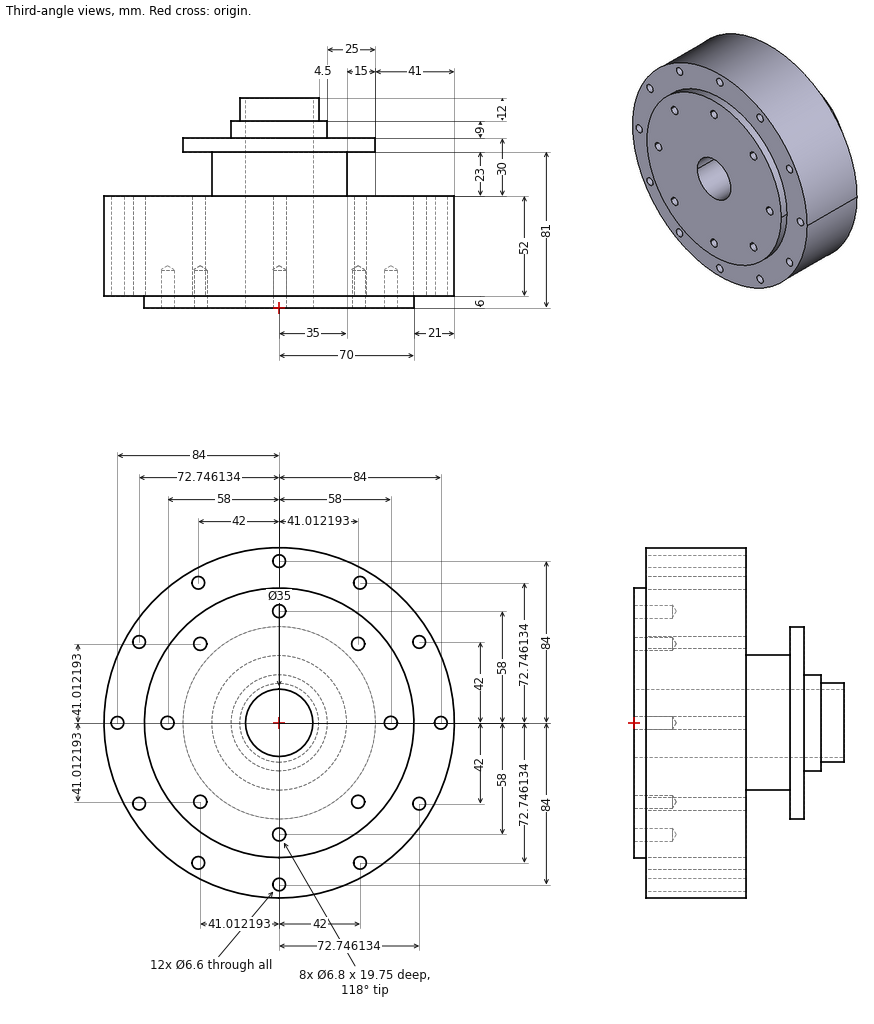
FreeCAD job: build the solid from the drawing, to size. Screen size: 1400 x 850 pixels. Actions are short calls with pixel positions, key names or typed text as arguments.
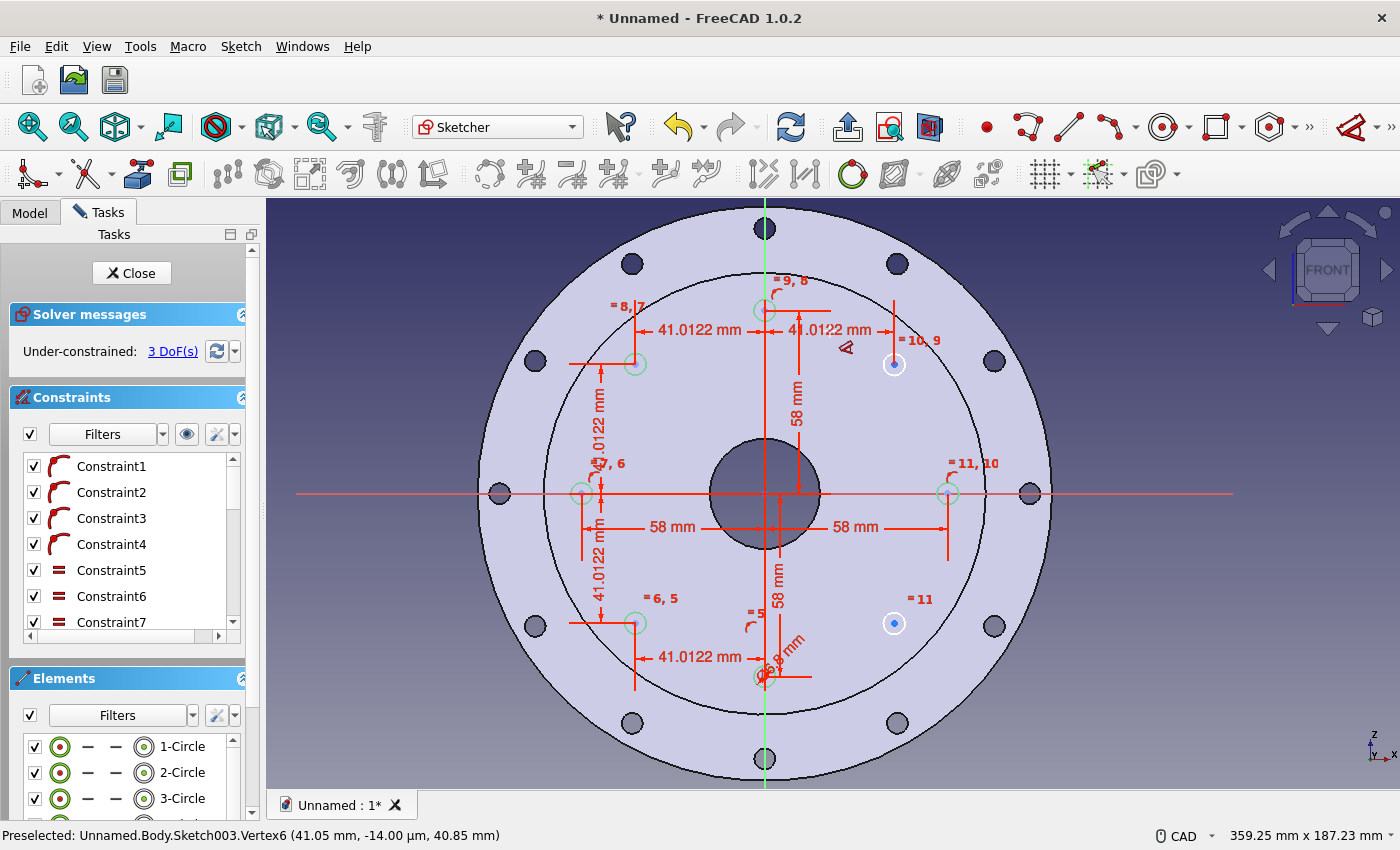
click(894, 365)
click(928, 429)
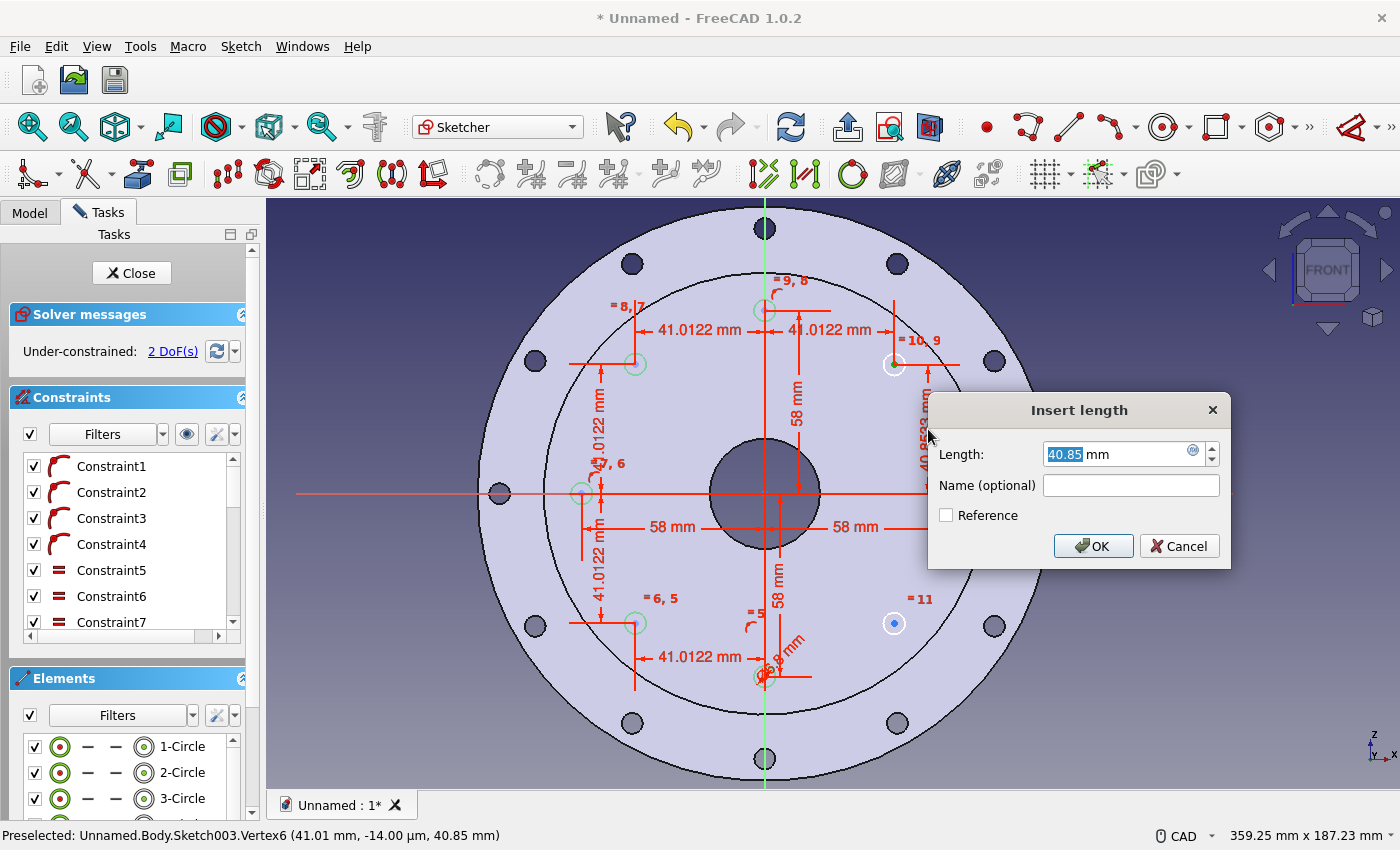
text(41.012193)
key(Return)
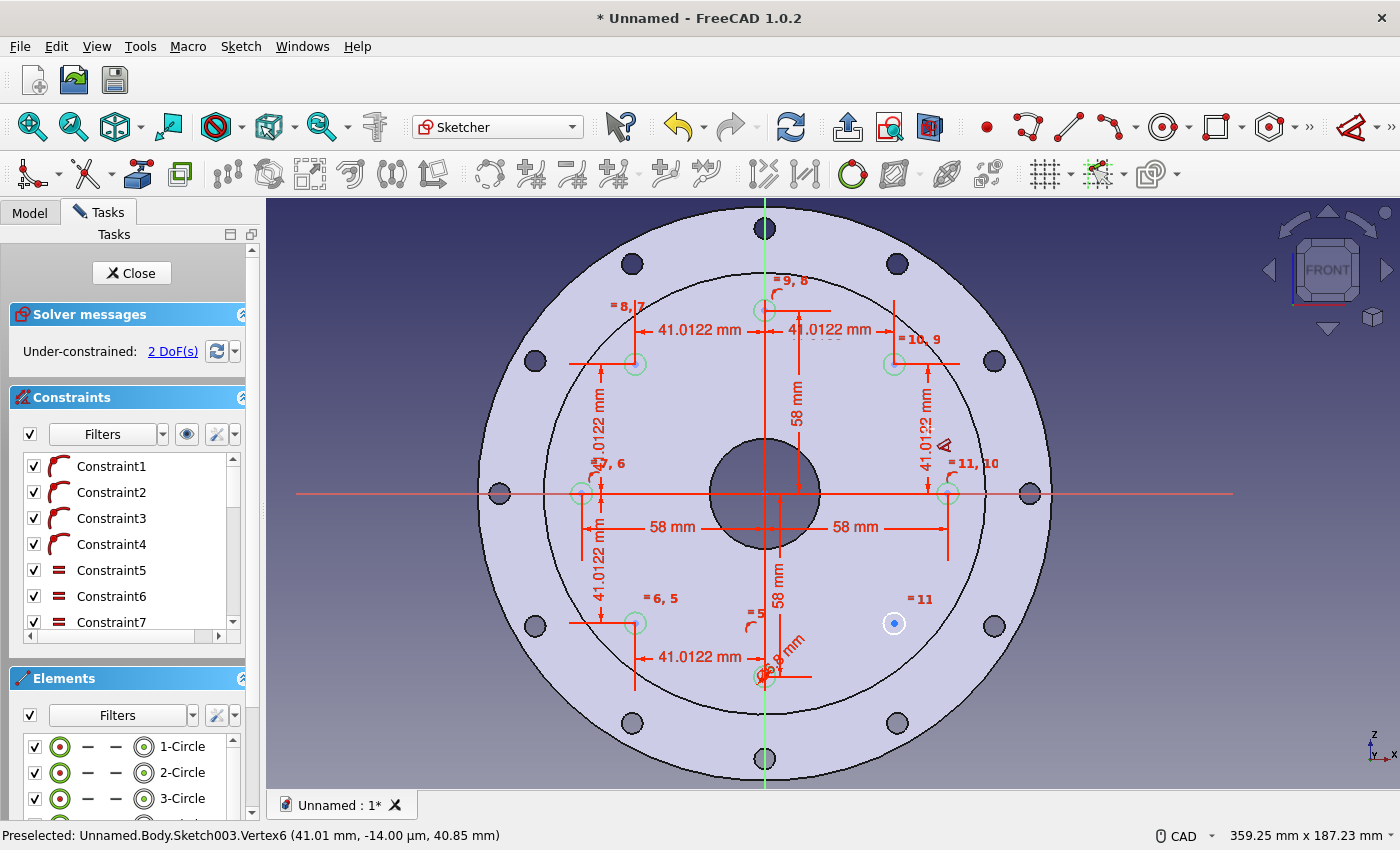
click(894, 624)
click(859, 658)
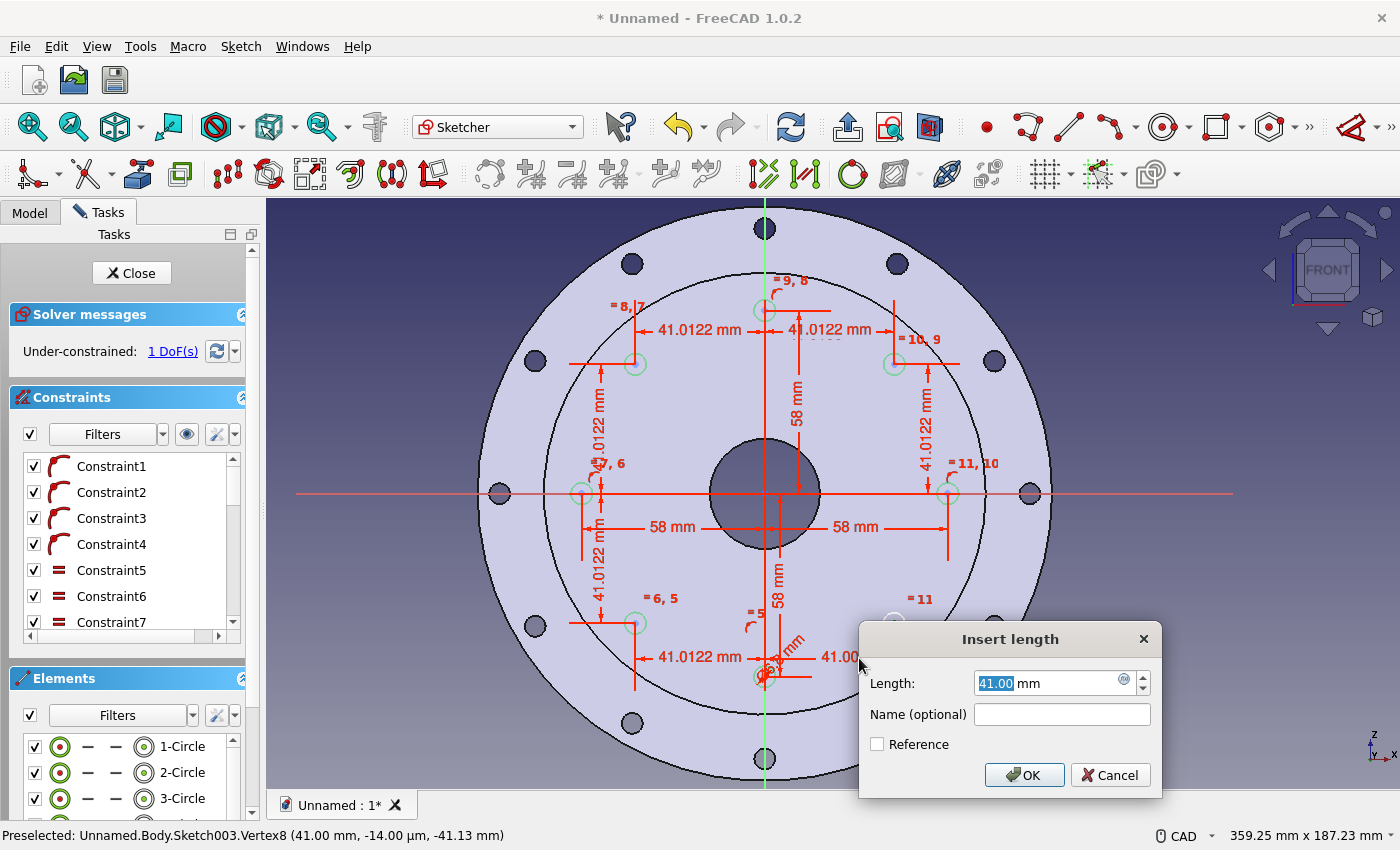
text(41.012193)
key(Return)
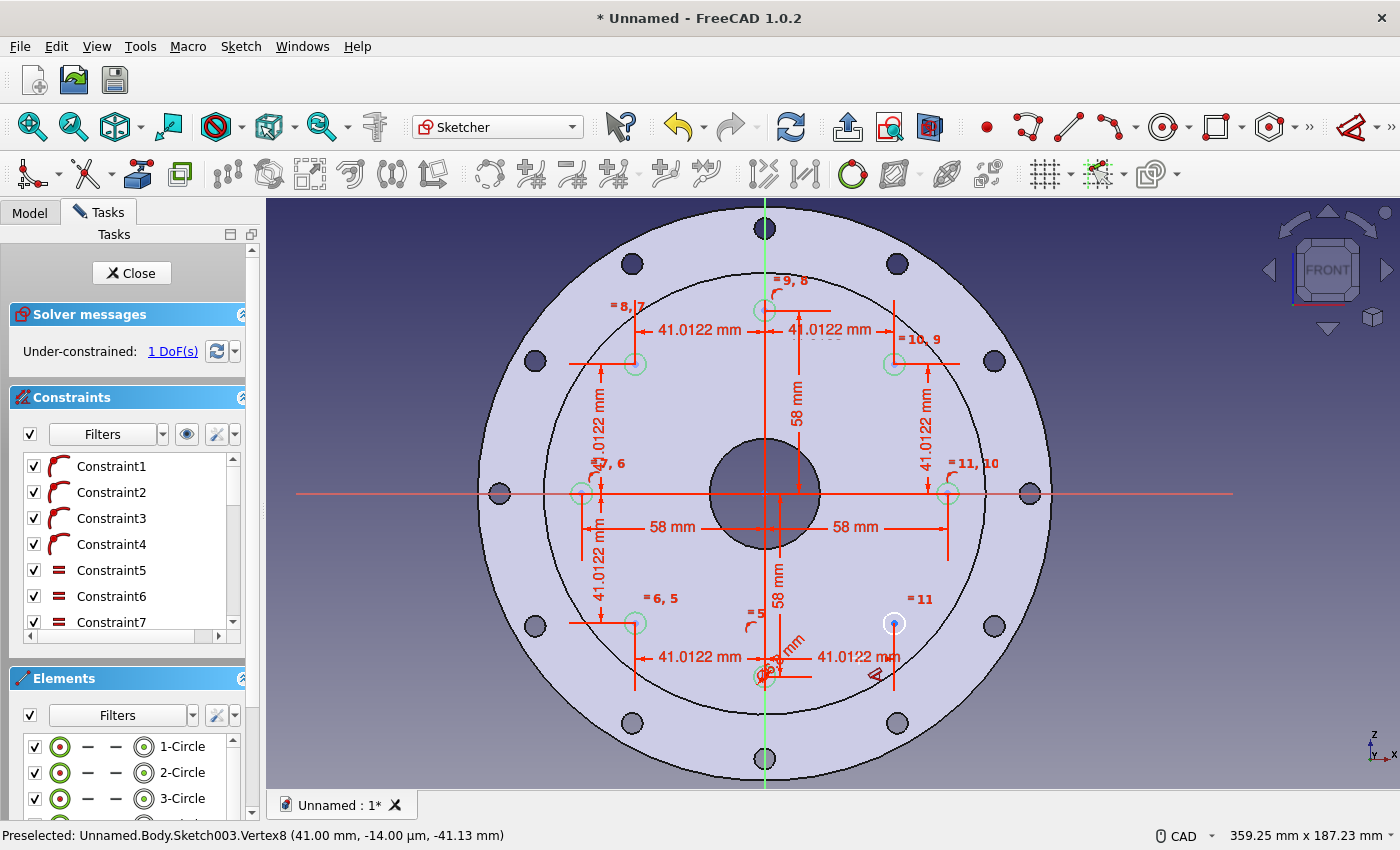
click(894, 624)
click(928, 559)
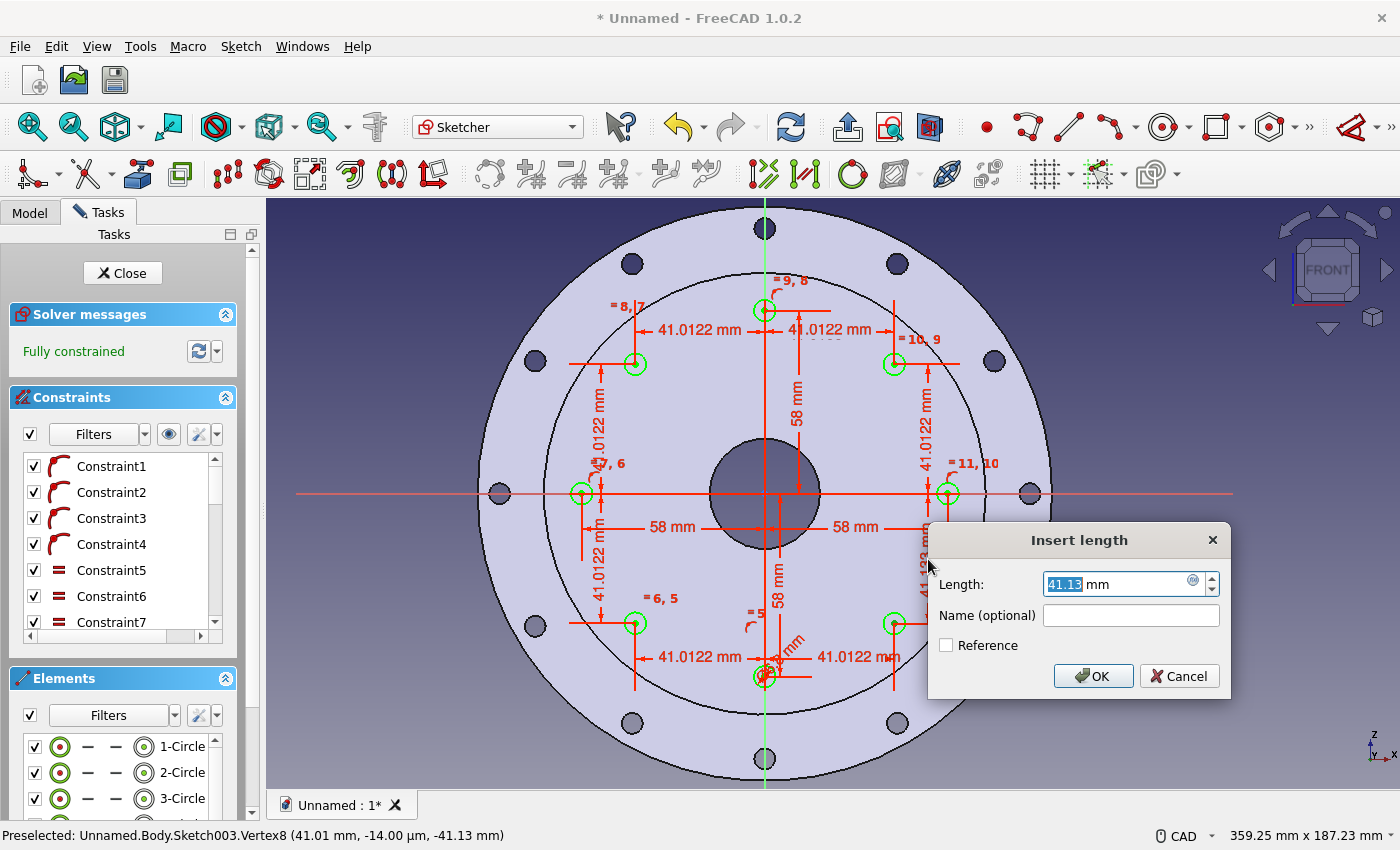
text(41.012193)
key(Return)
key(Escape)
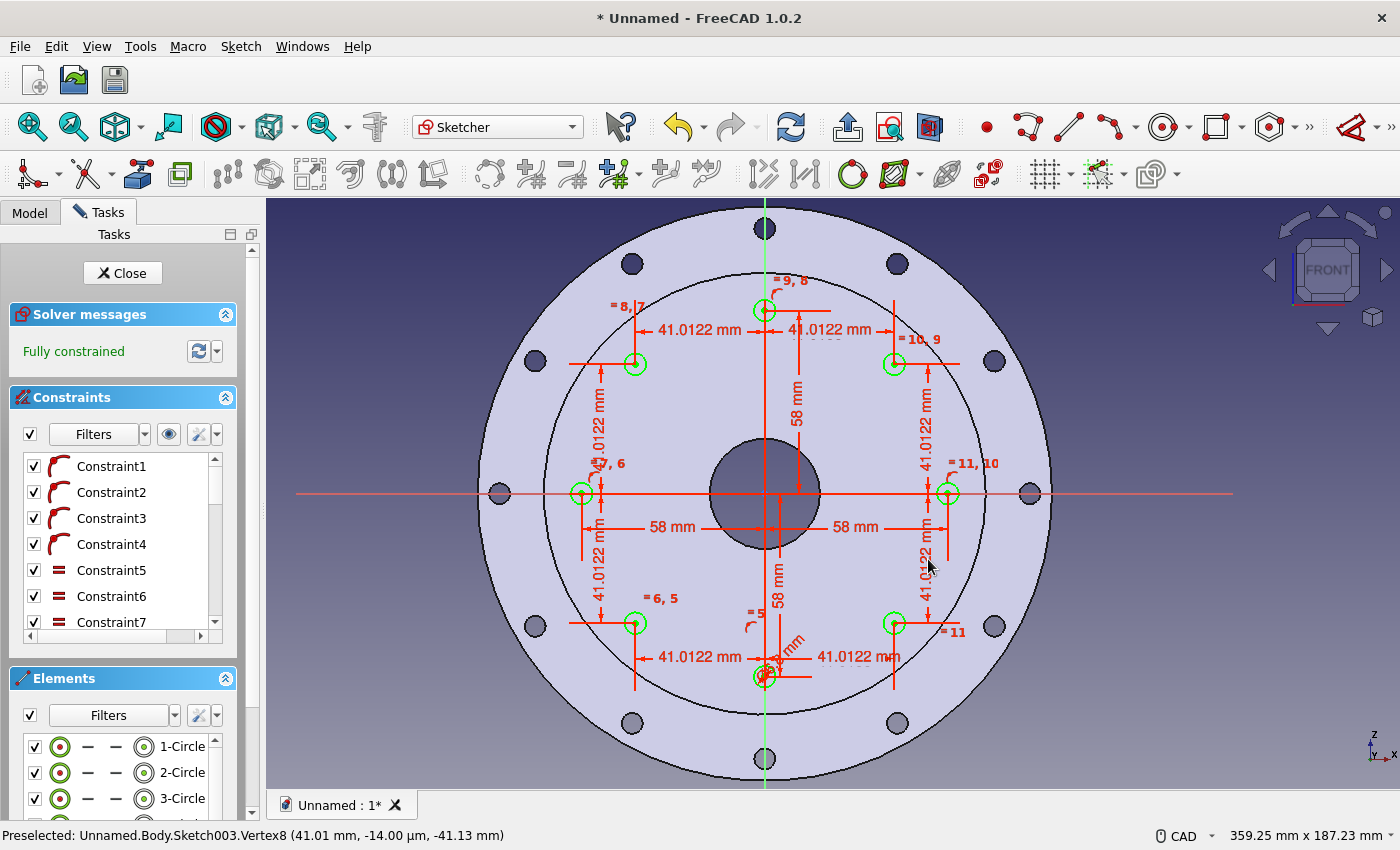
click(123, 273)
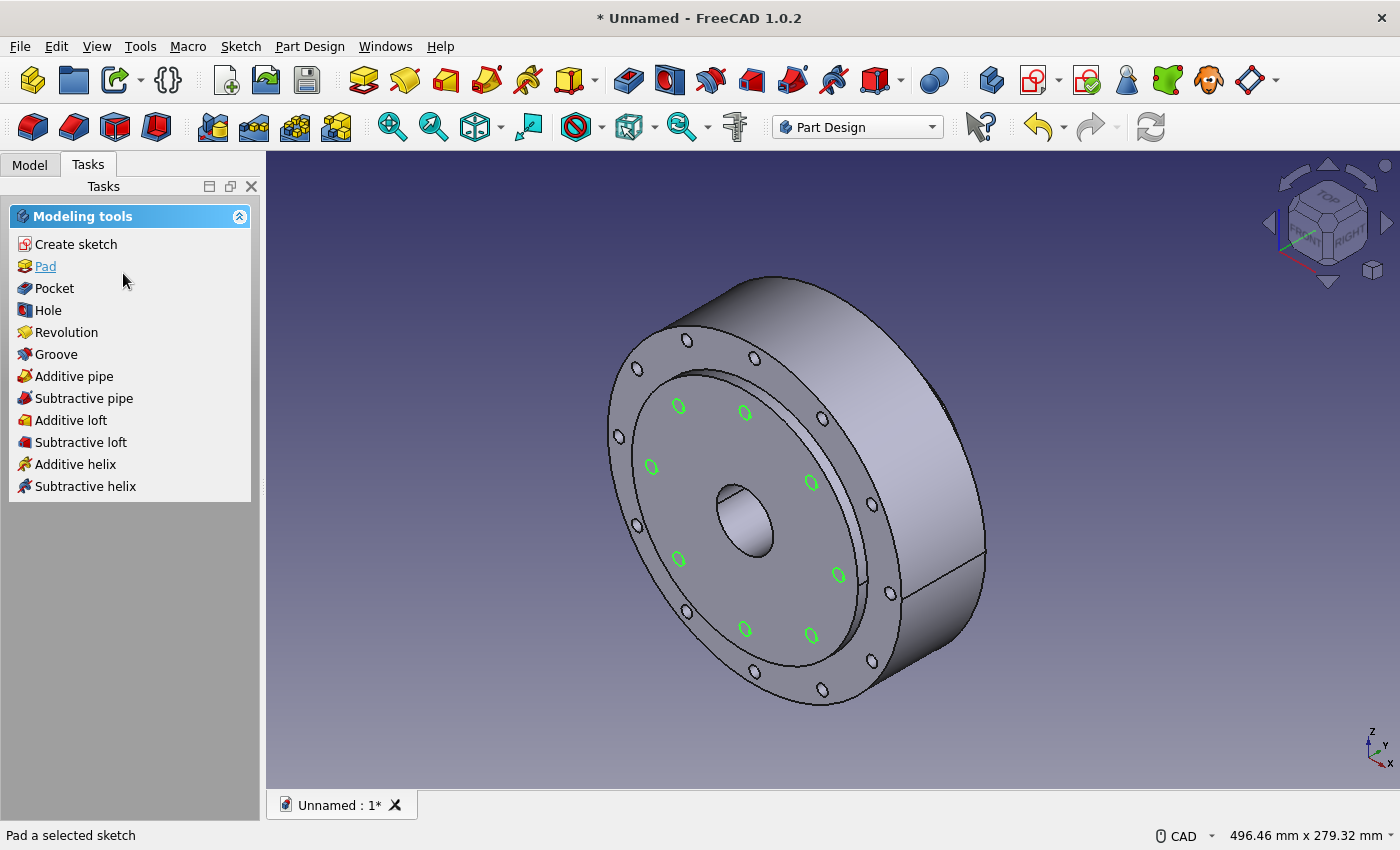
click(670, 80)